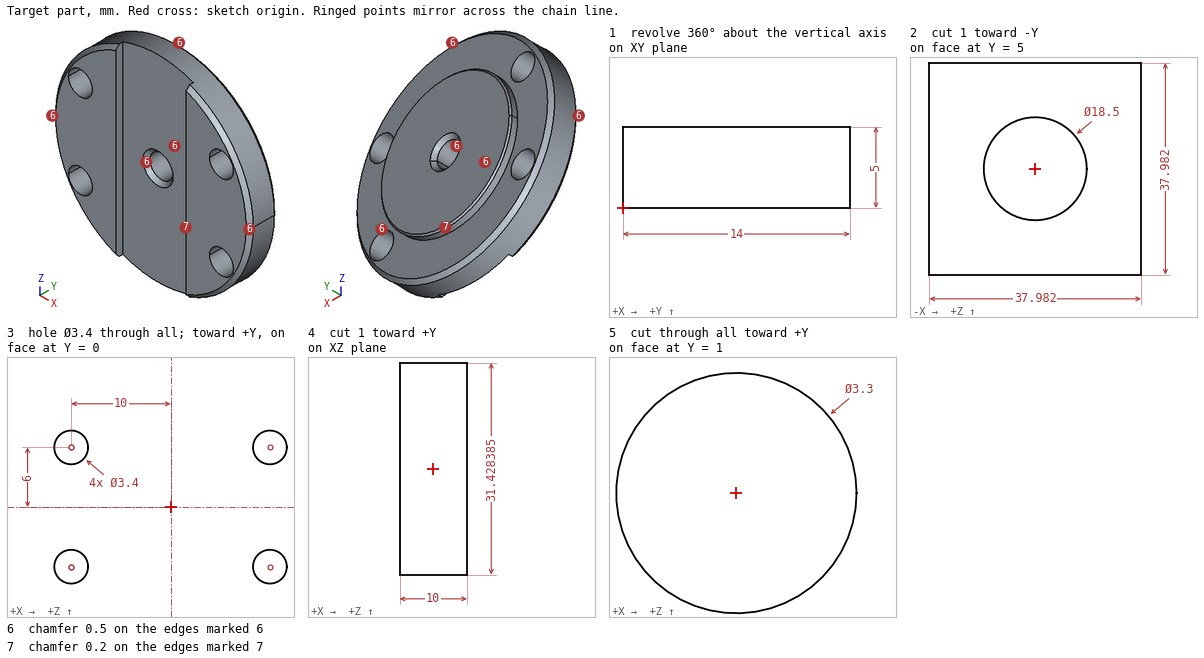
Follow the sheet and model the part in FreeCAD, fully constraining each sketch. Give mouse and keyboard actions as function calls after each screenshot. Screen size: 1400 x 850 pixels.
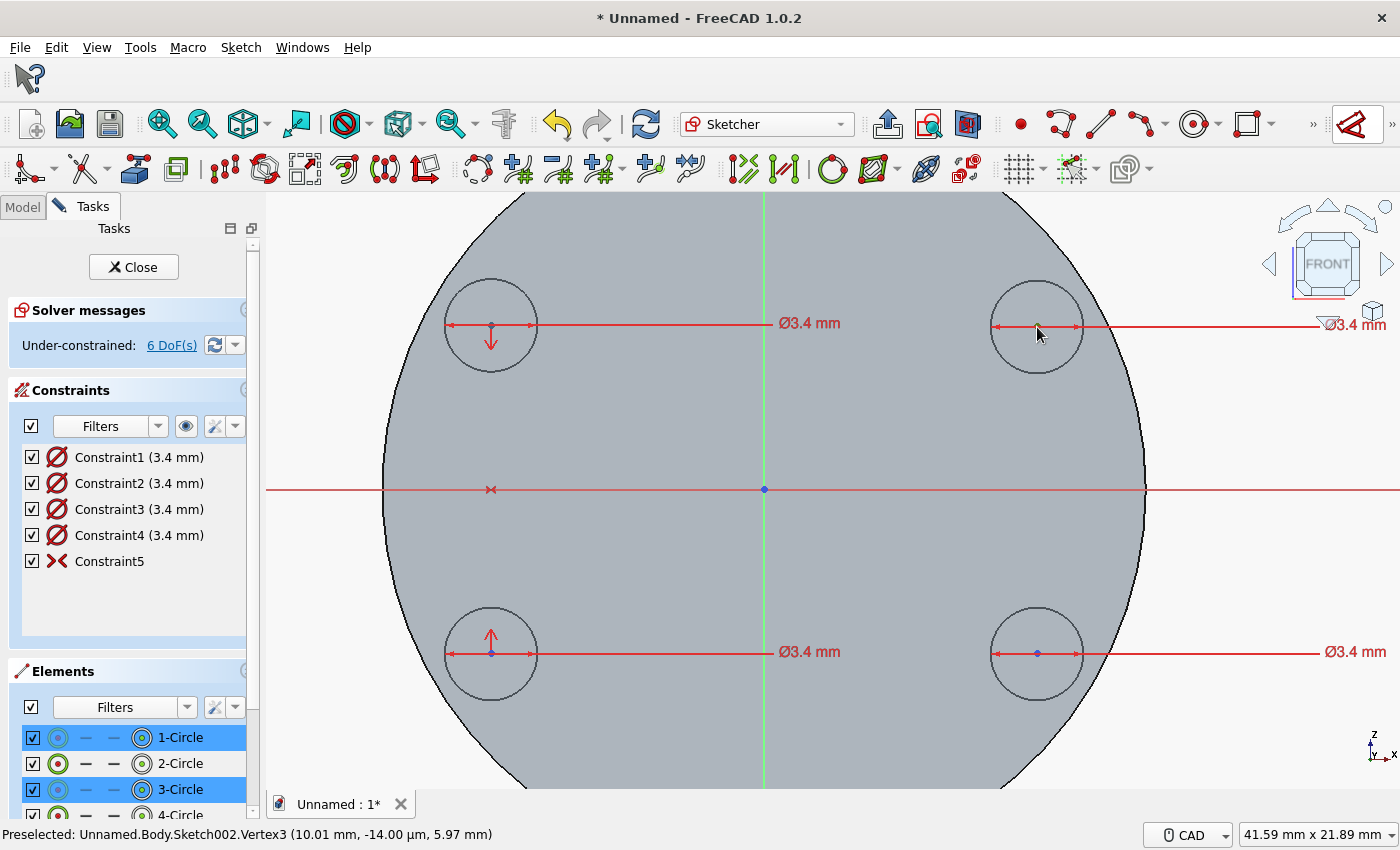
click(764, 722)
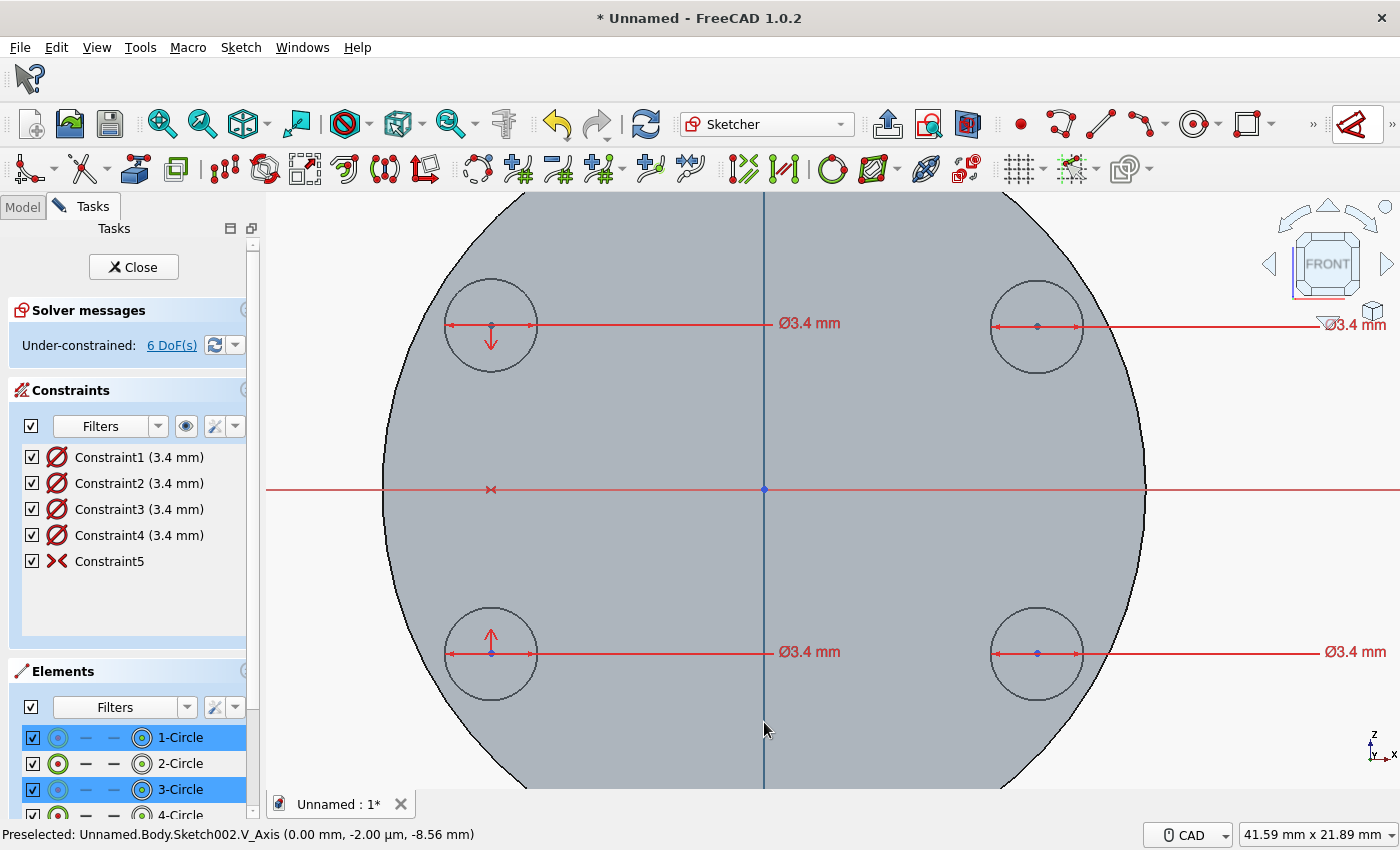
key(s)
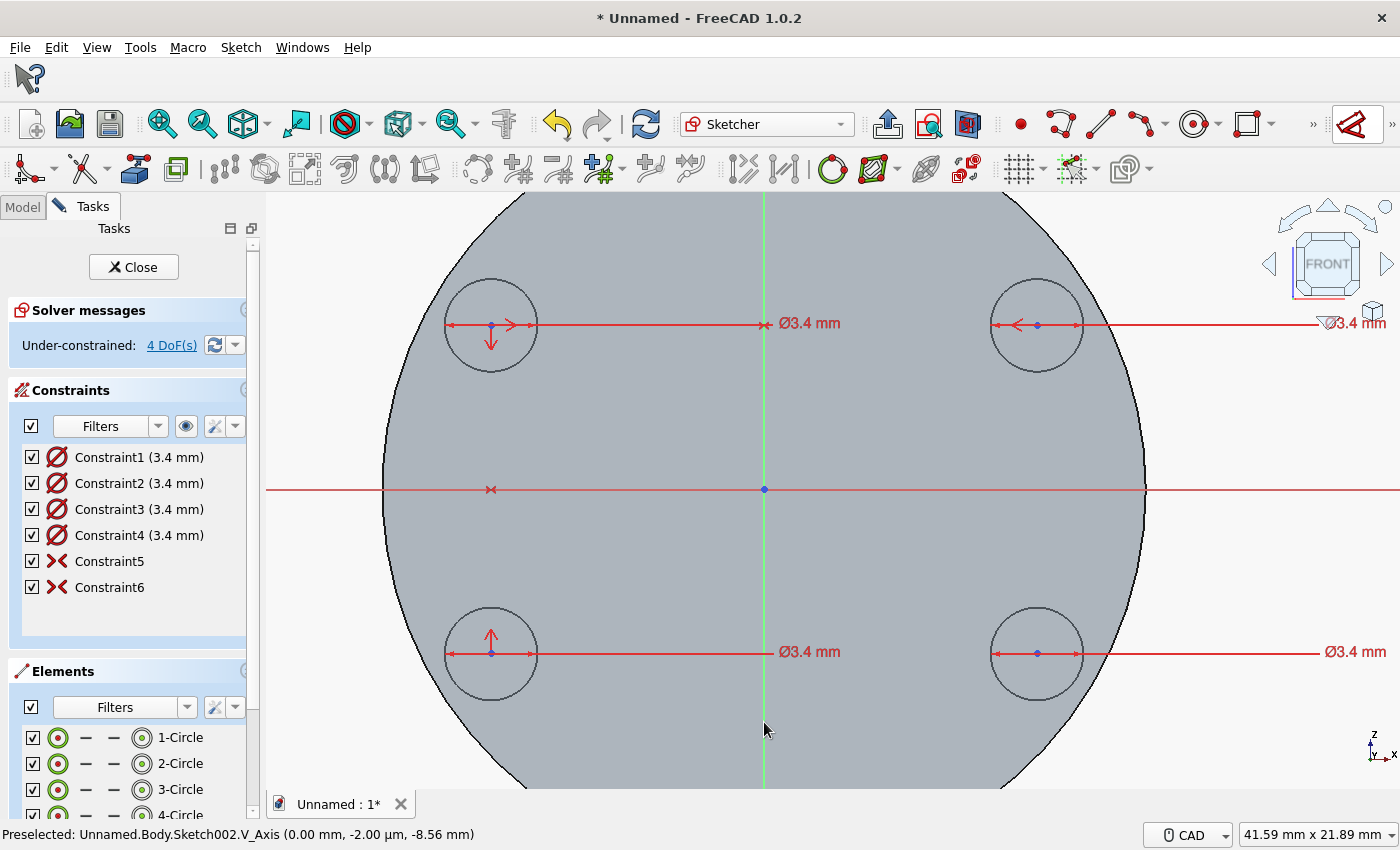
click(491, 654)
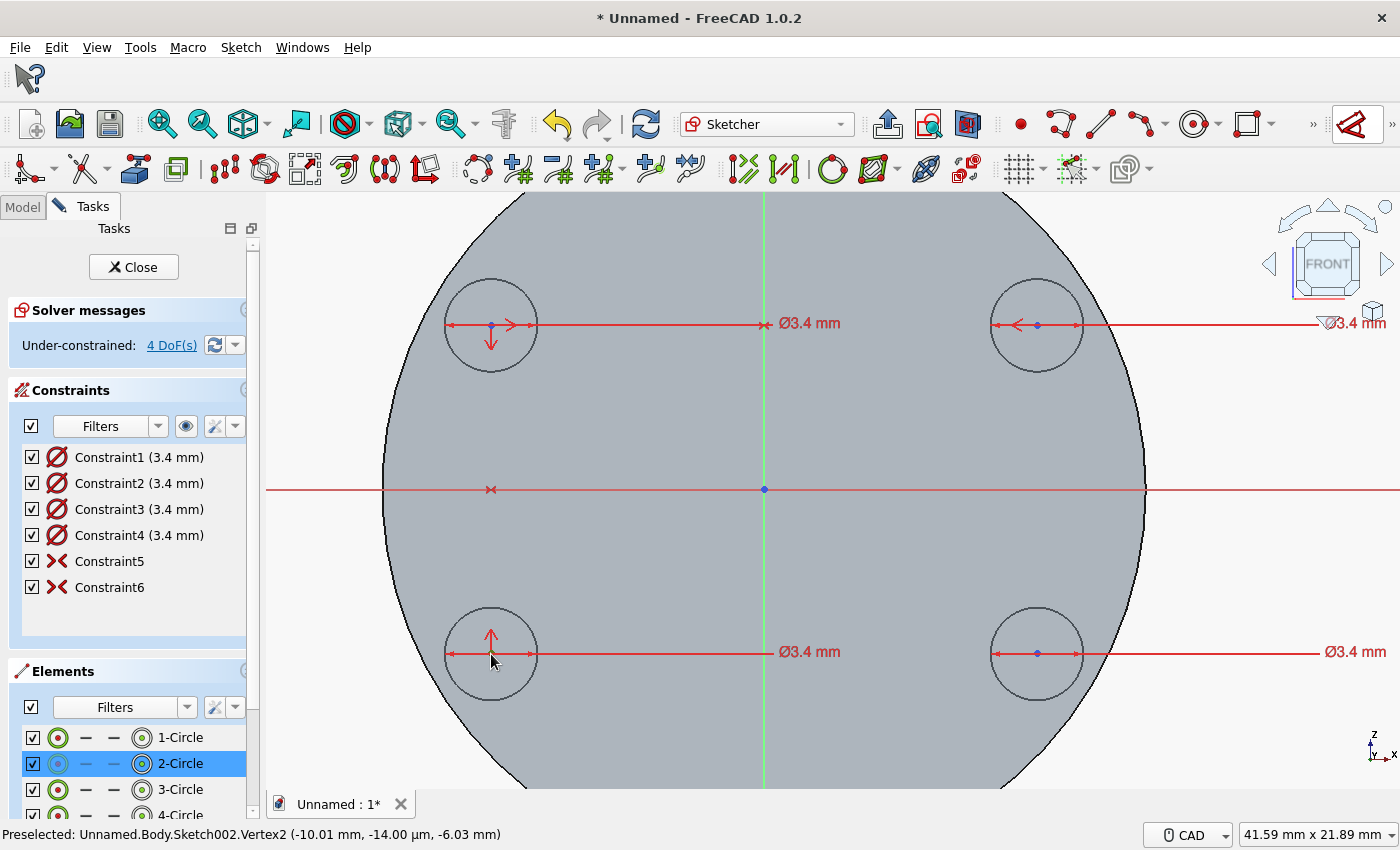
click(1037, 654)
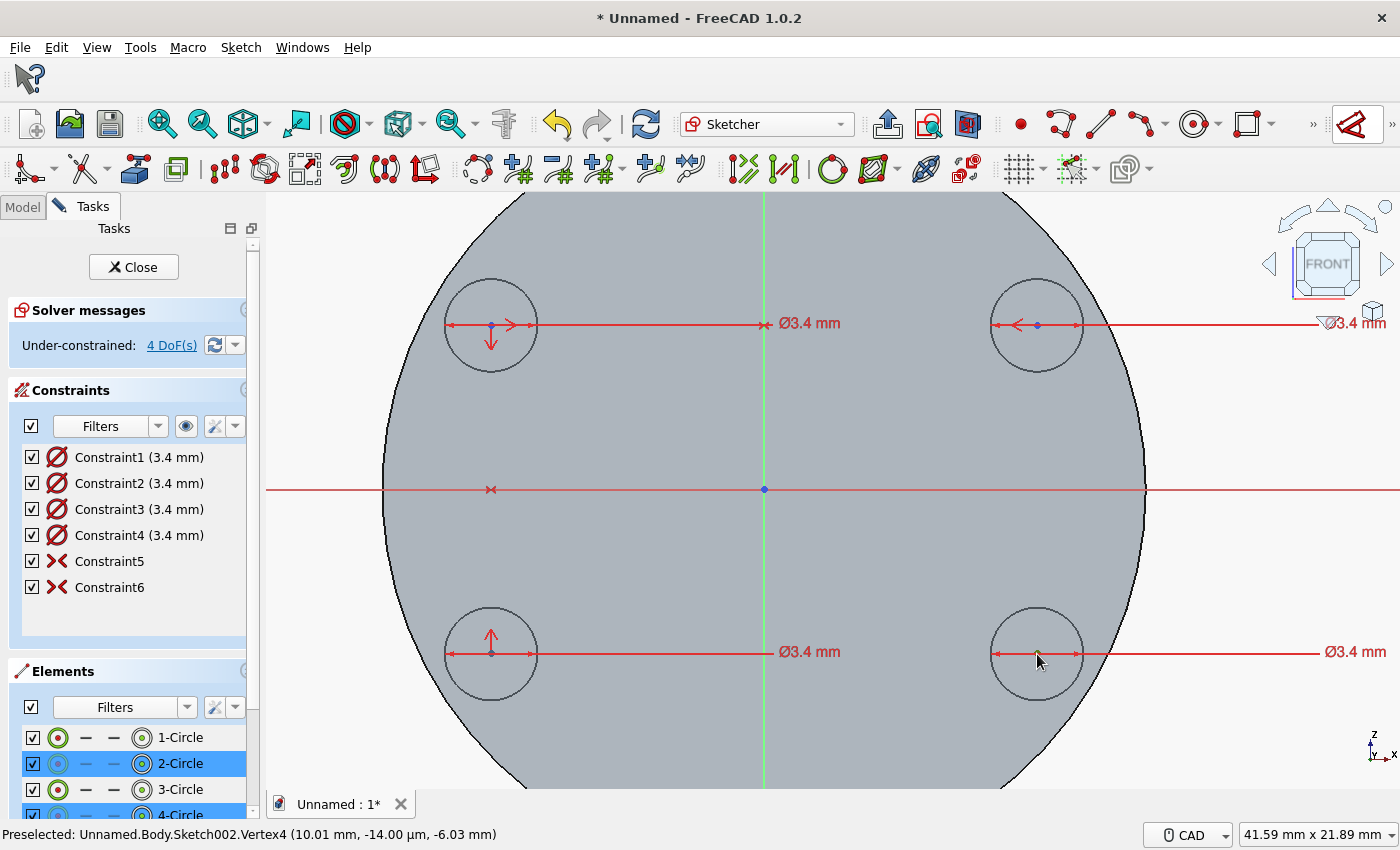
click(764, 722)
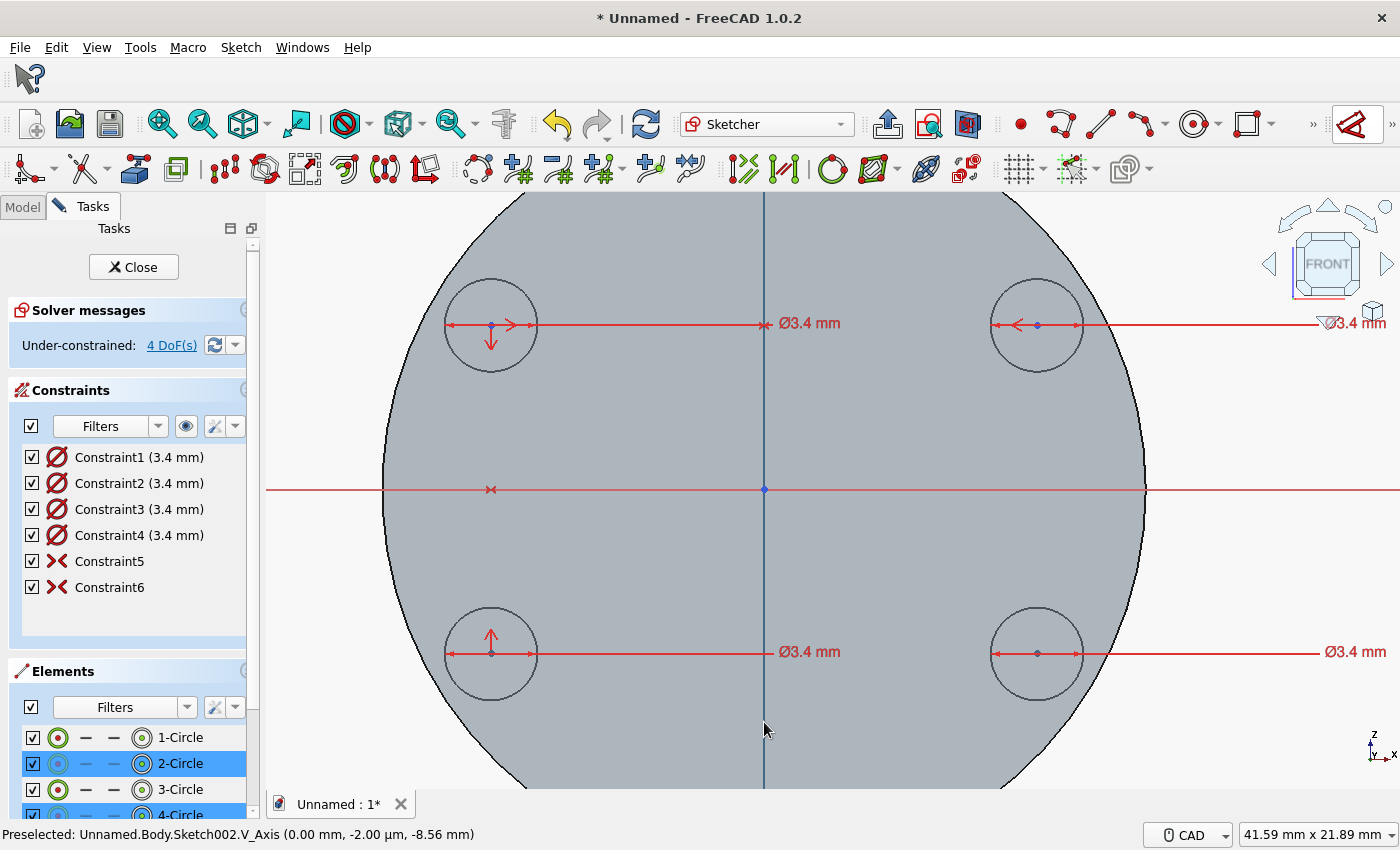
key(s)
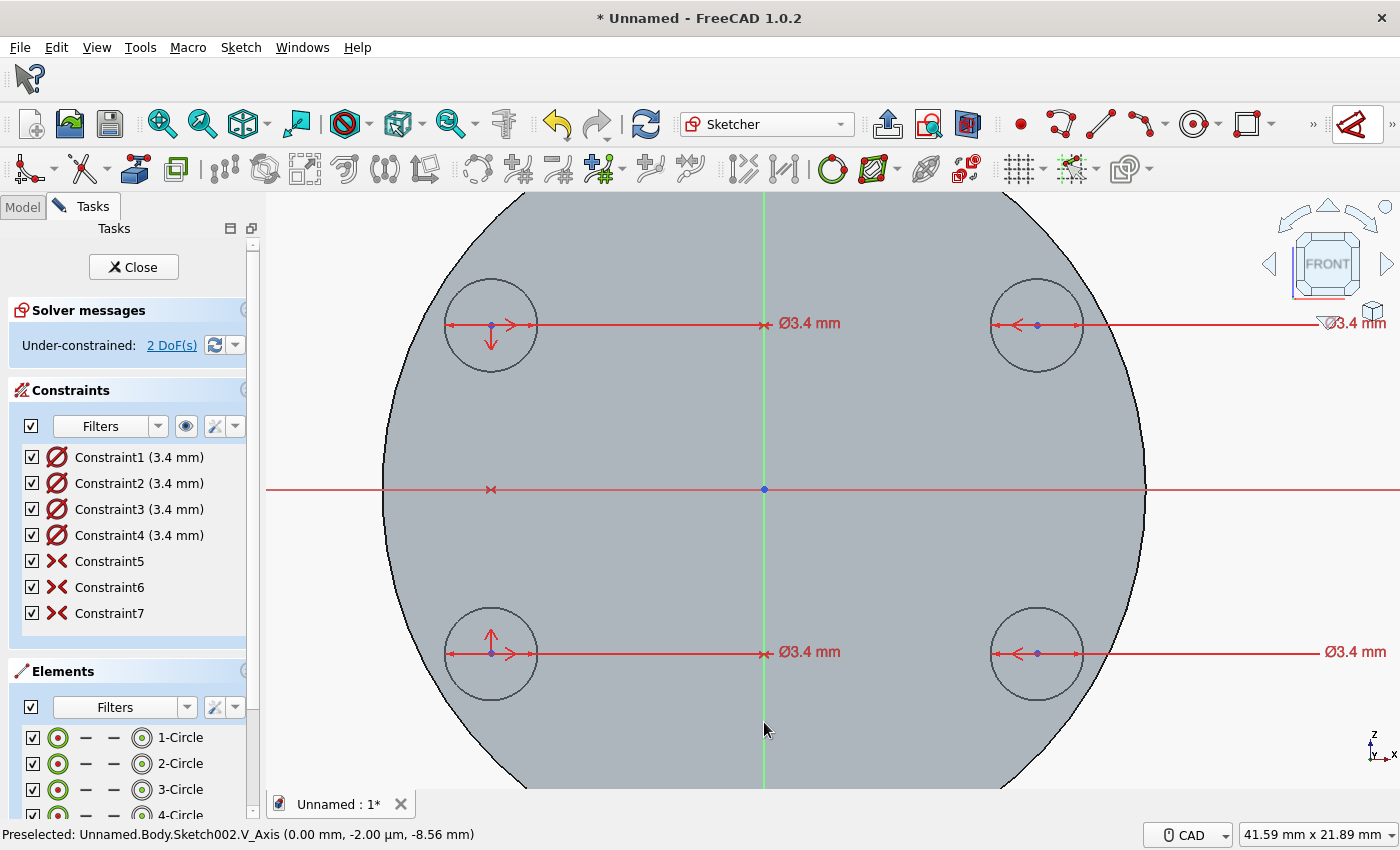
click(491, 325)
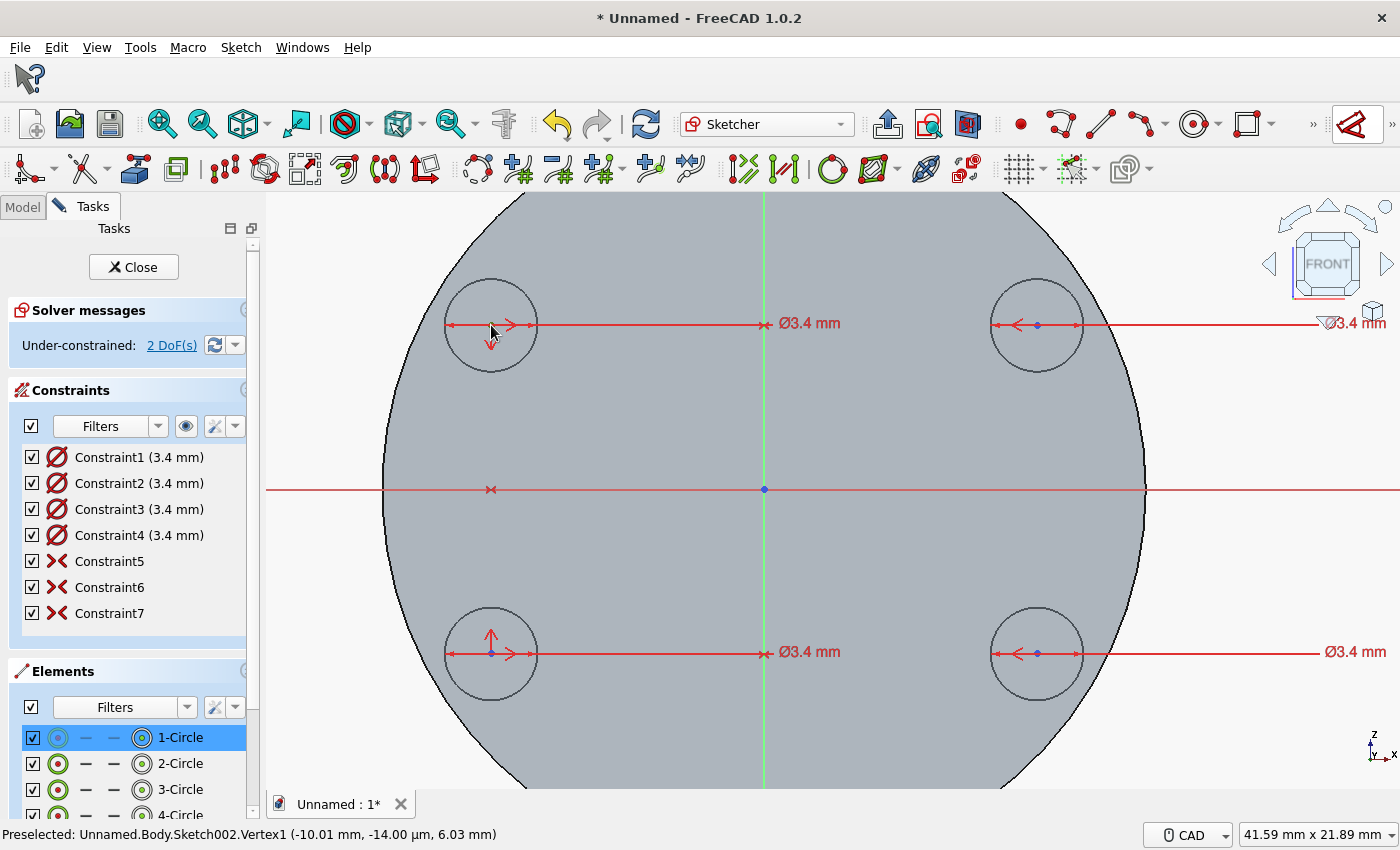
key(i)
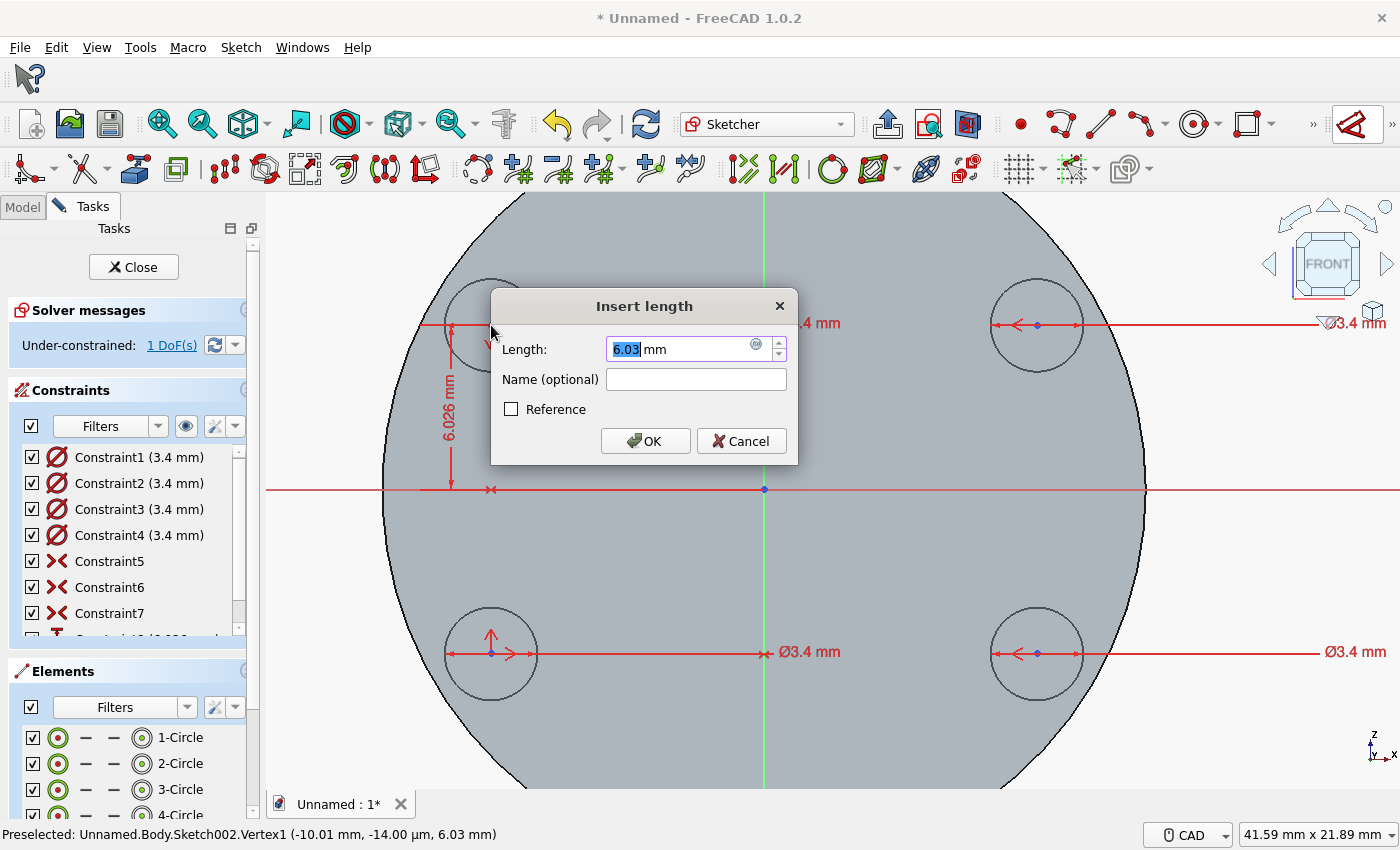
text(6)
key(Return)